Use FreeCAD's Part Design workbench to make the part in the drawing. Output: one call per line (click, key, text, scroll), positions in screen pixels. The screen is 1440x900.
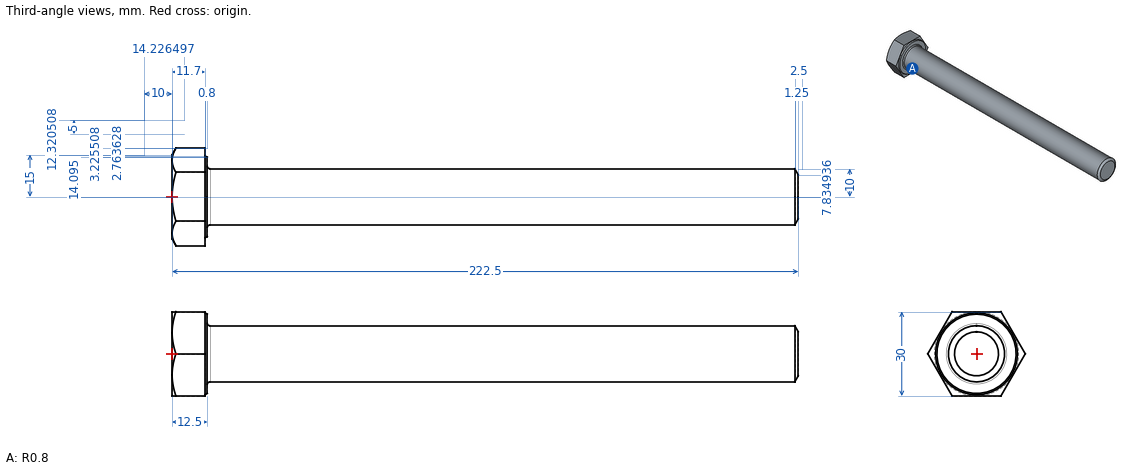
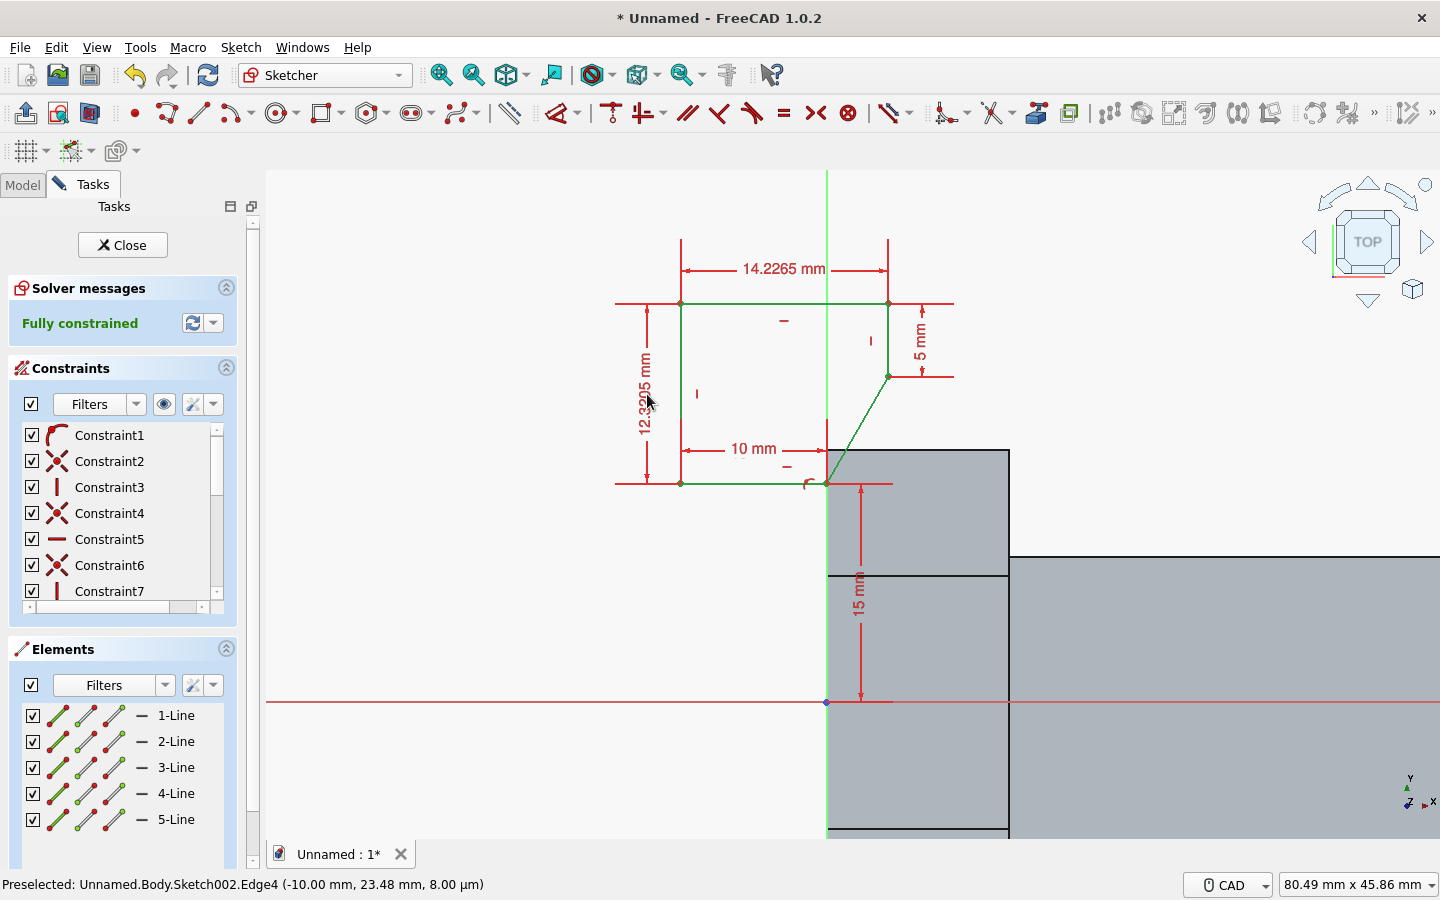
click(123, 245)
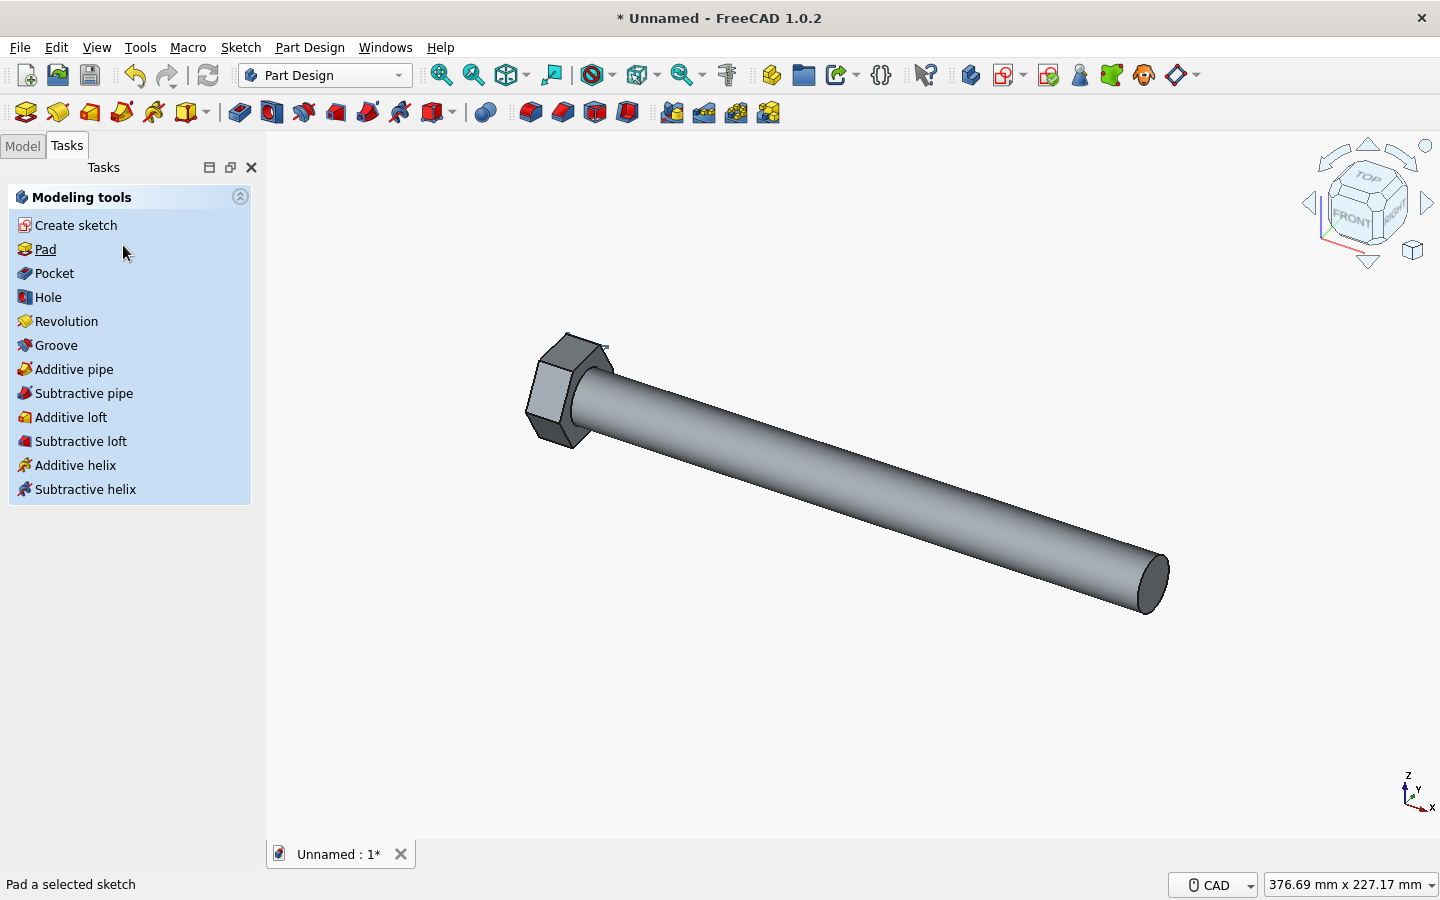
click(304, 112)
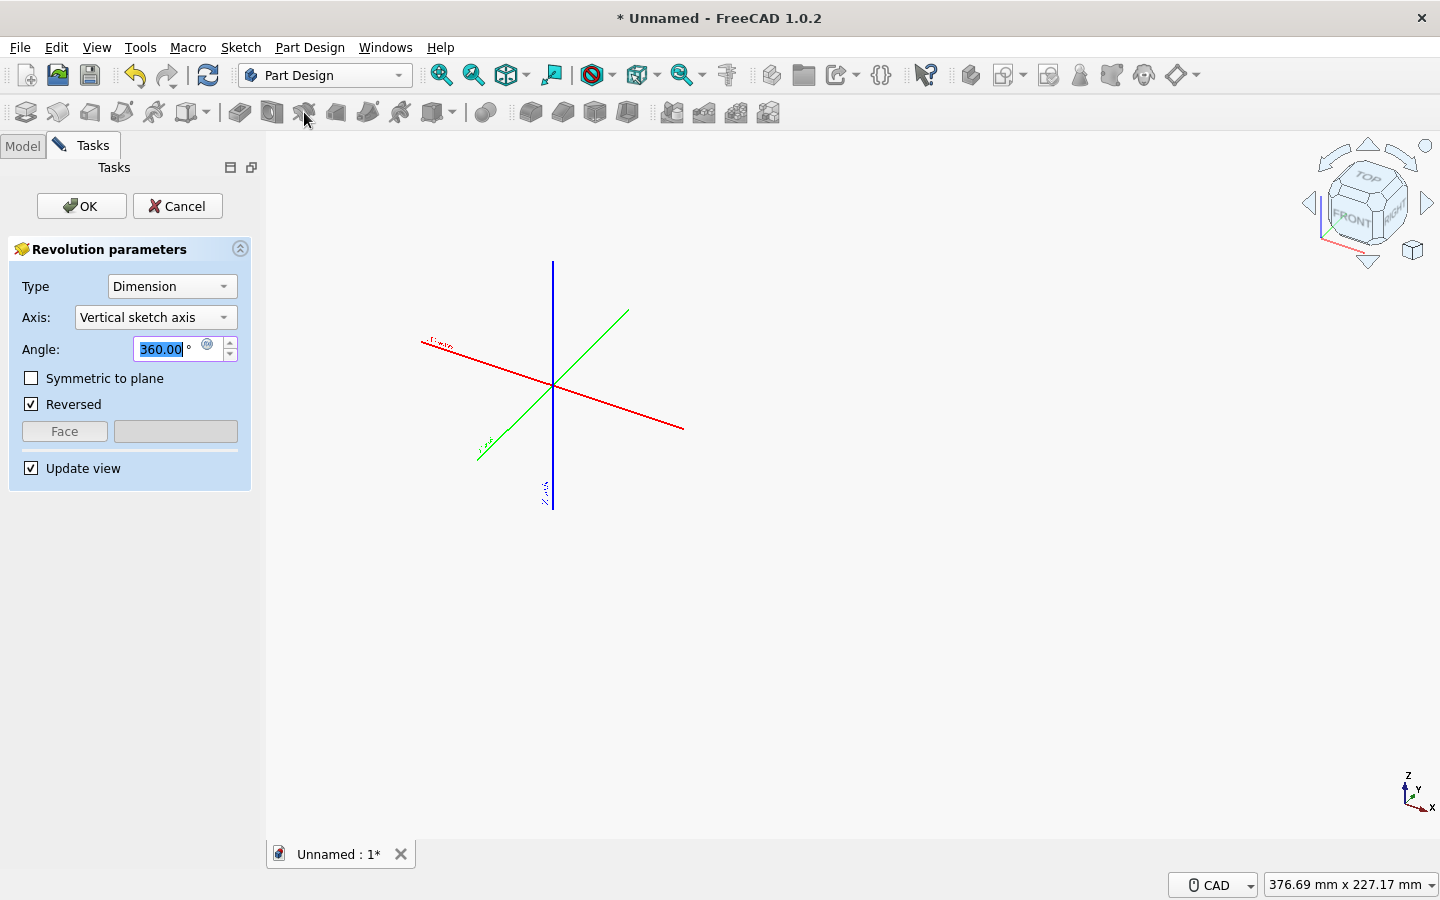
click(156, 318)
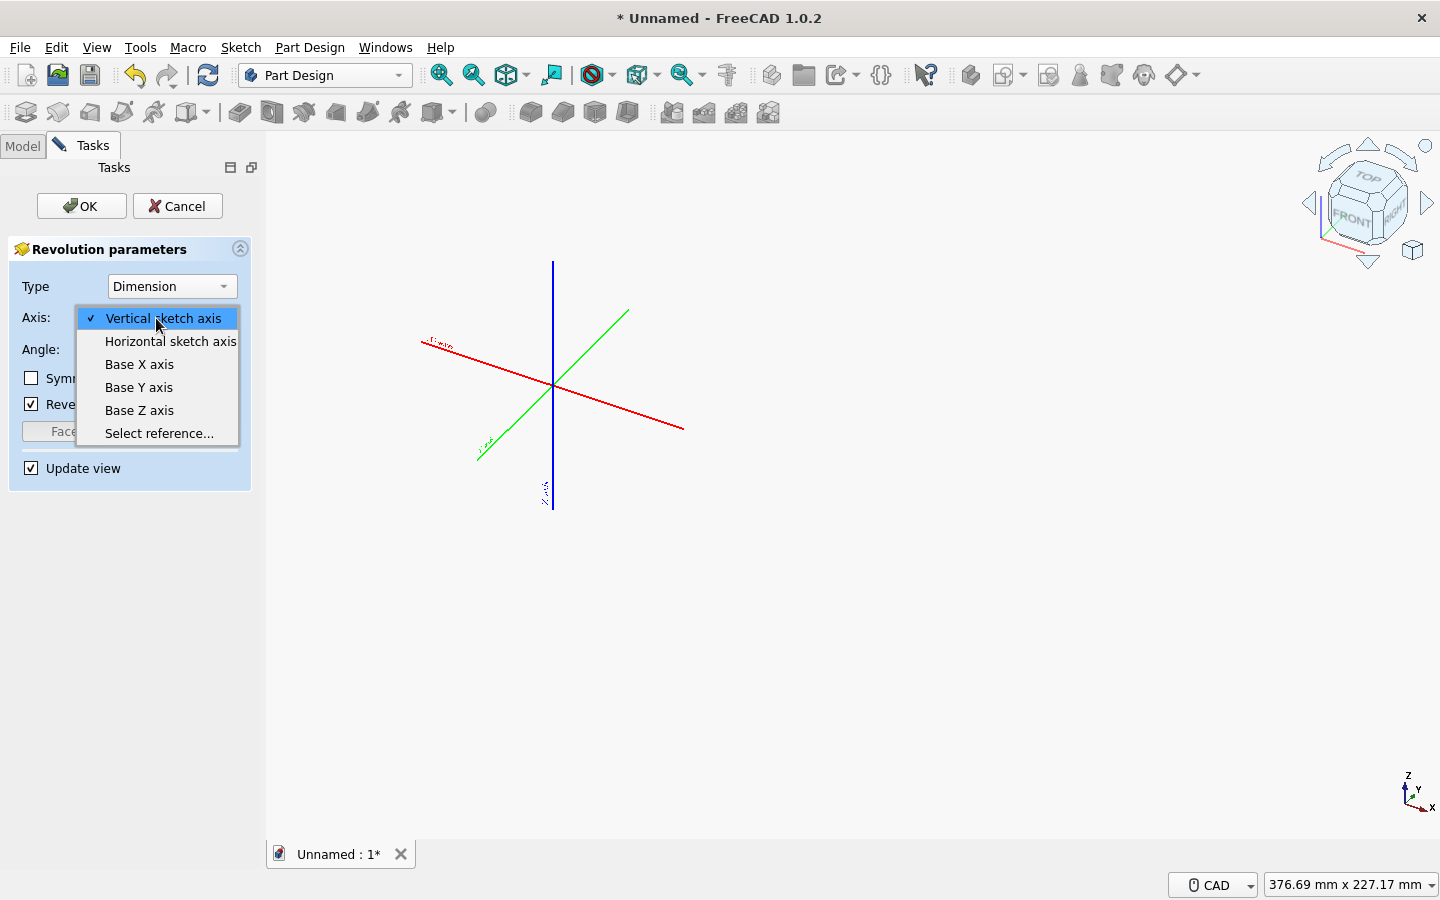
click(156, 342)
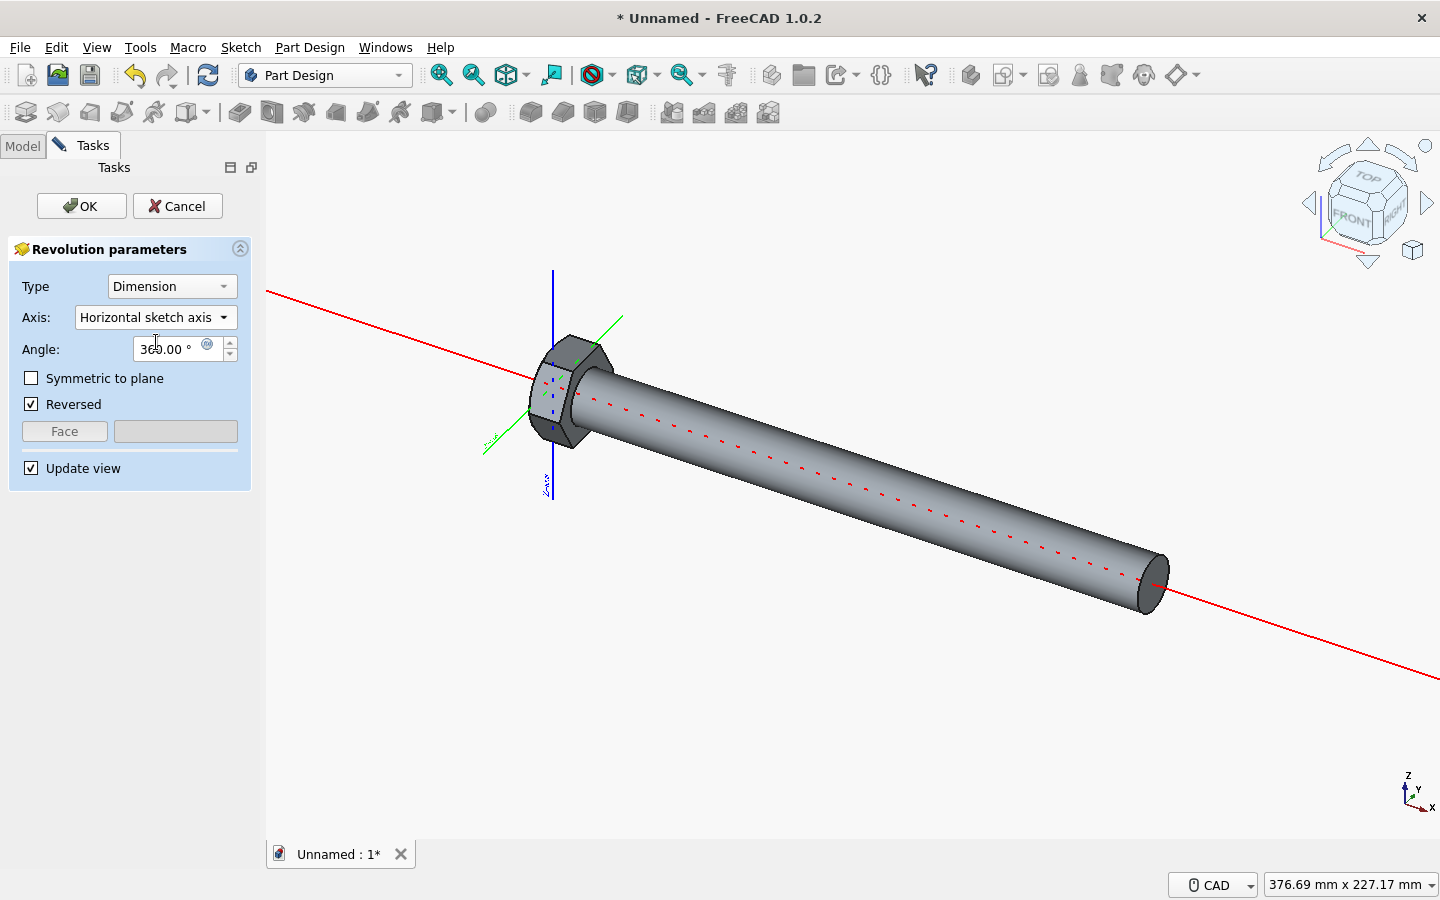
click(82, 206)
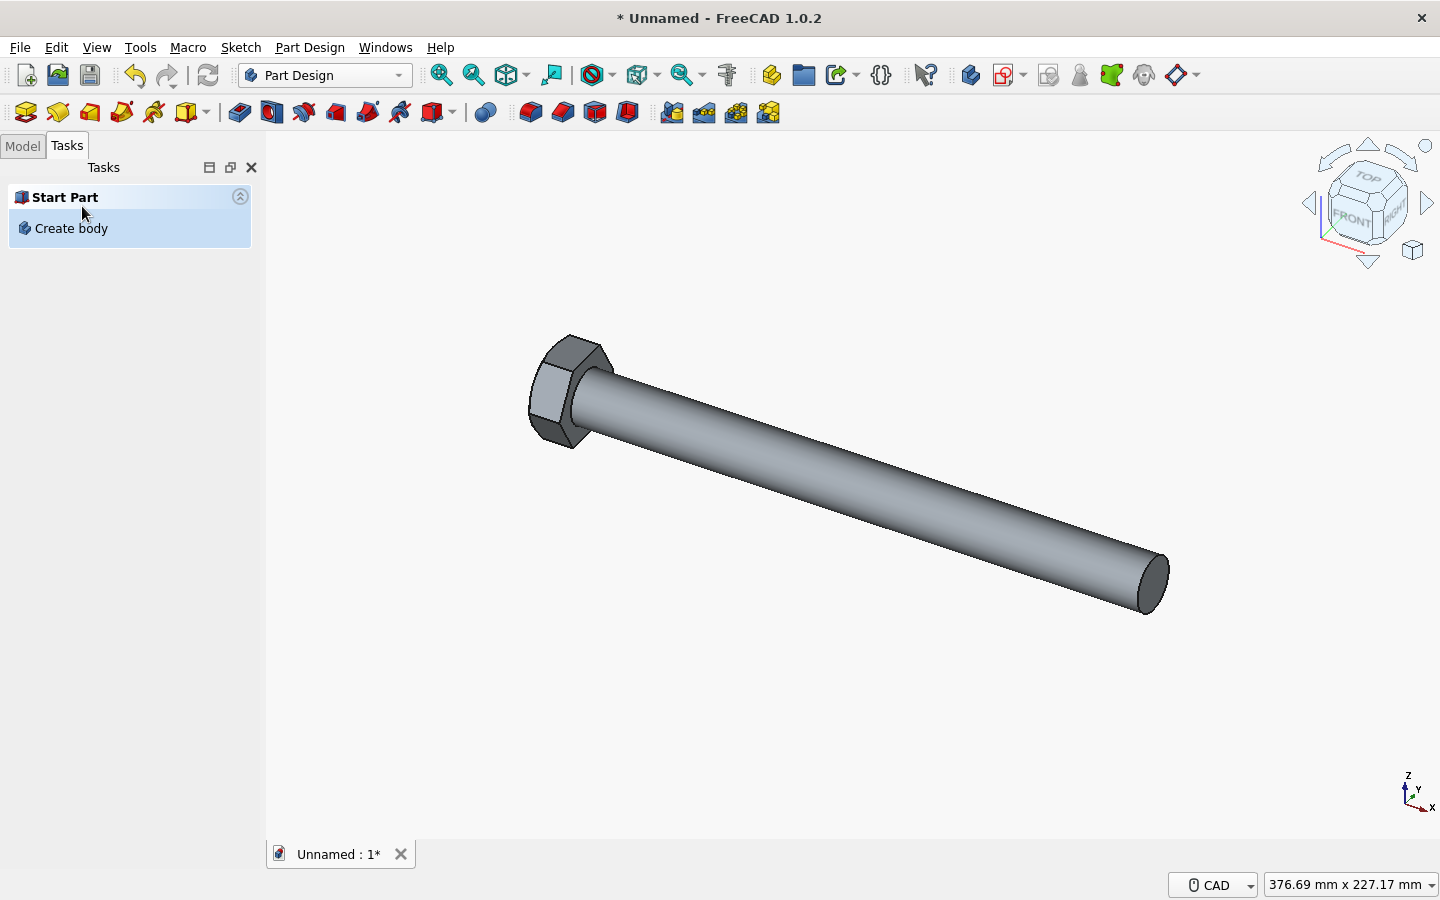
click(1004, 76)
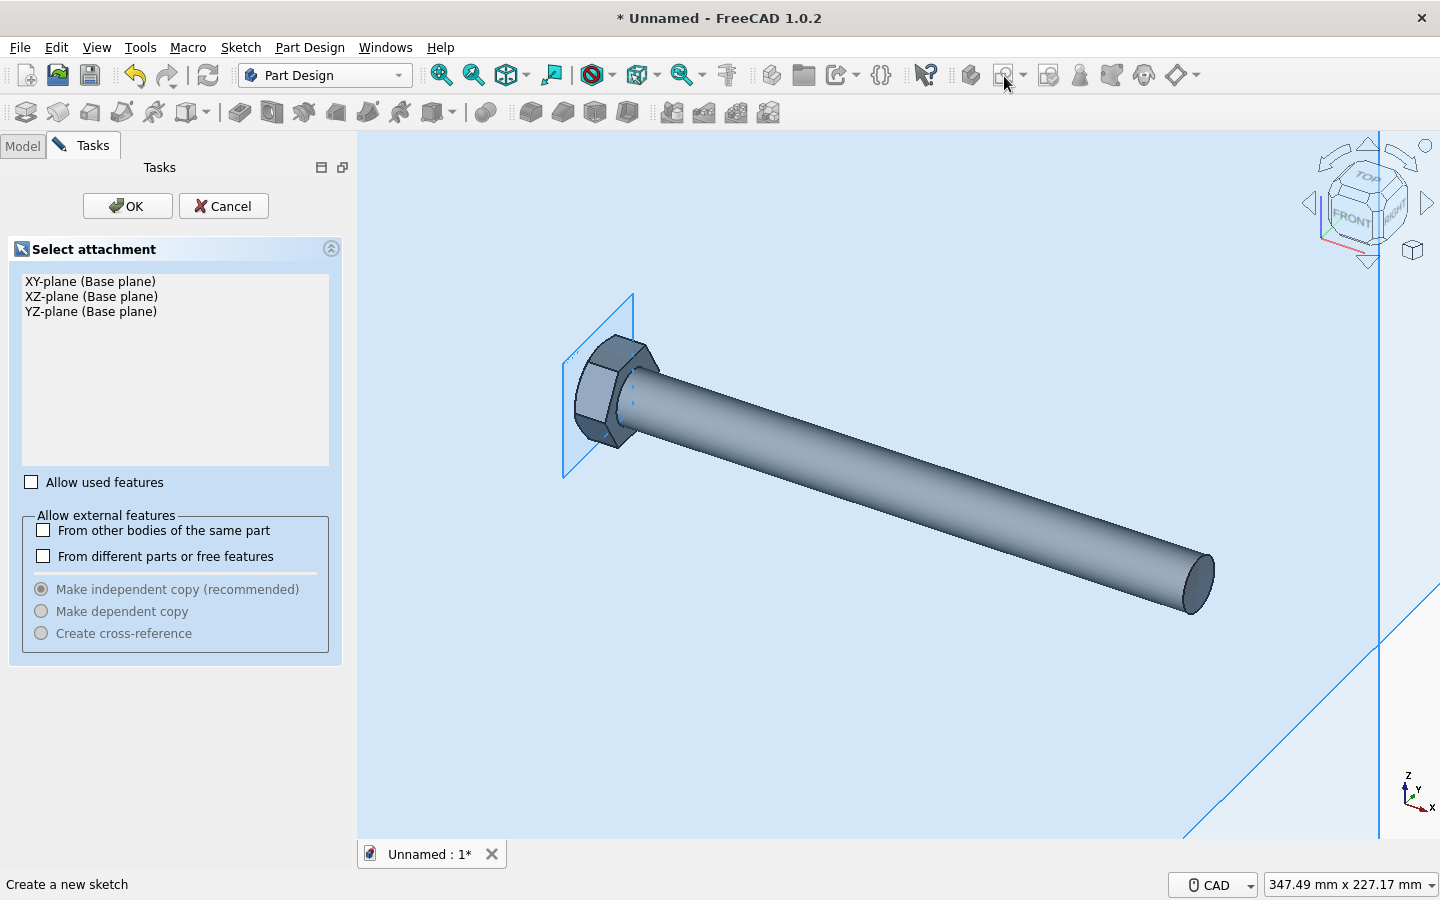
click(82, 282)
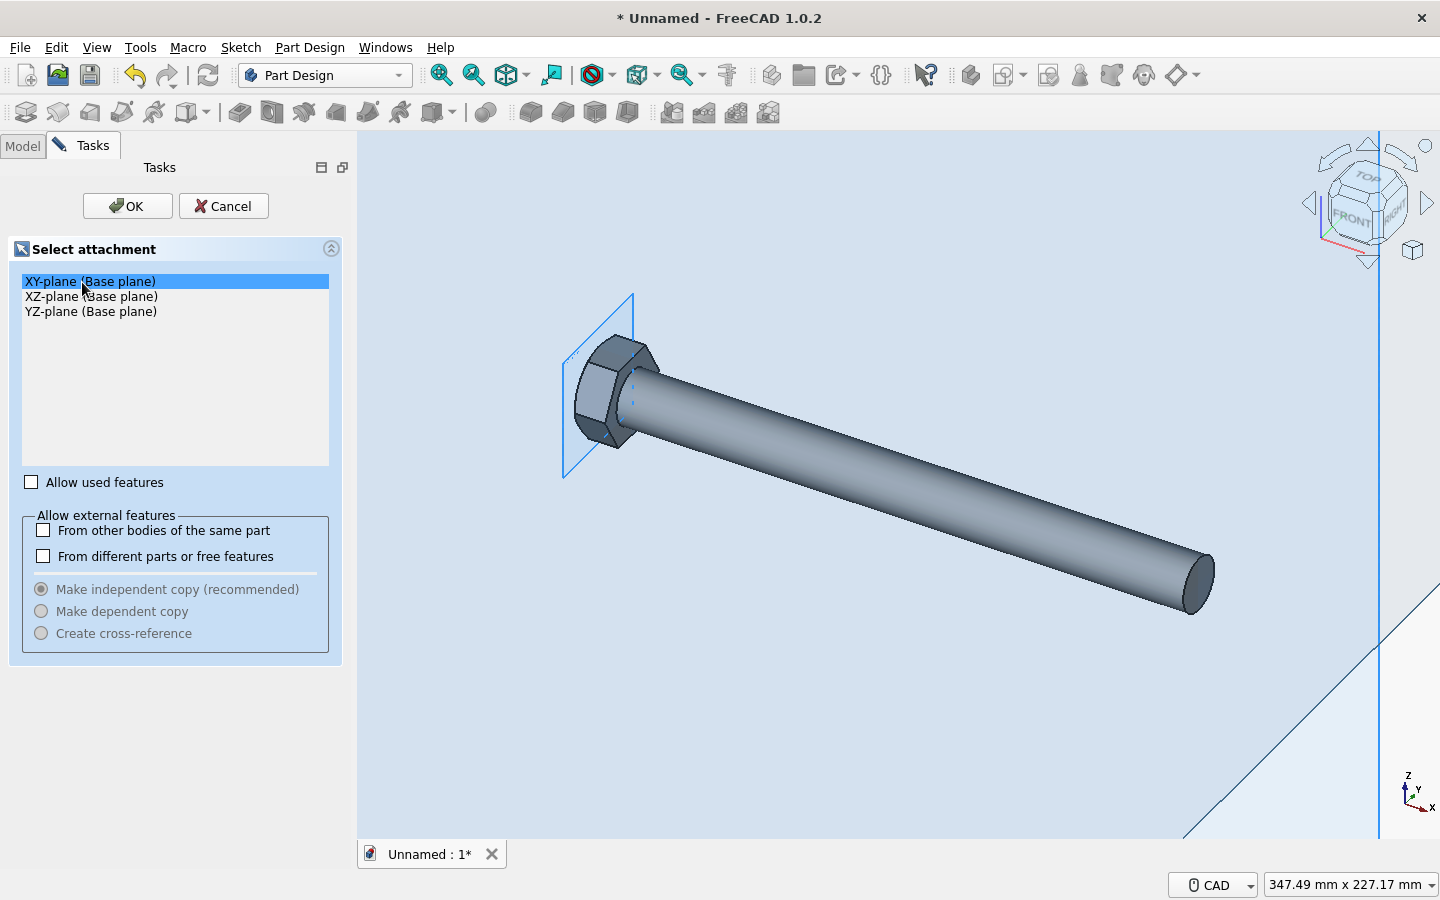
click(128, 206)